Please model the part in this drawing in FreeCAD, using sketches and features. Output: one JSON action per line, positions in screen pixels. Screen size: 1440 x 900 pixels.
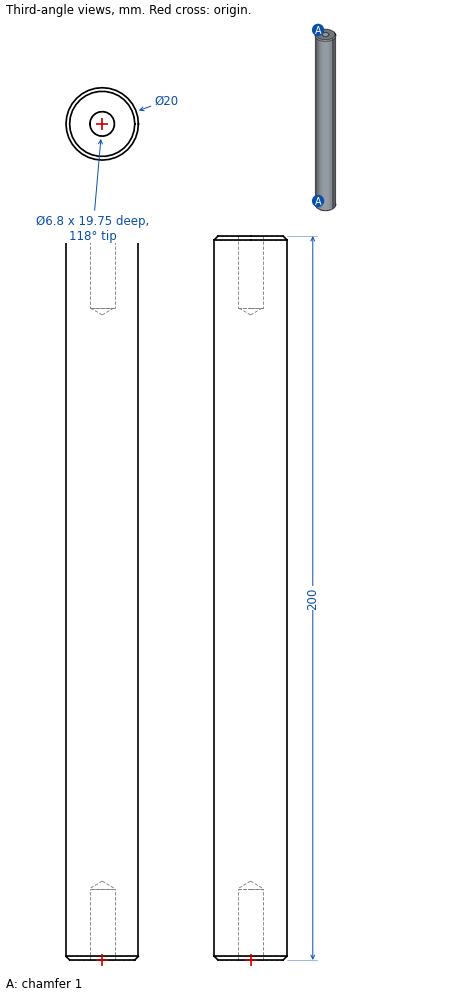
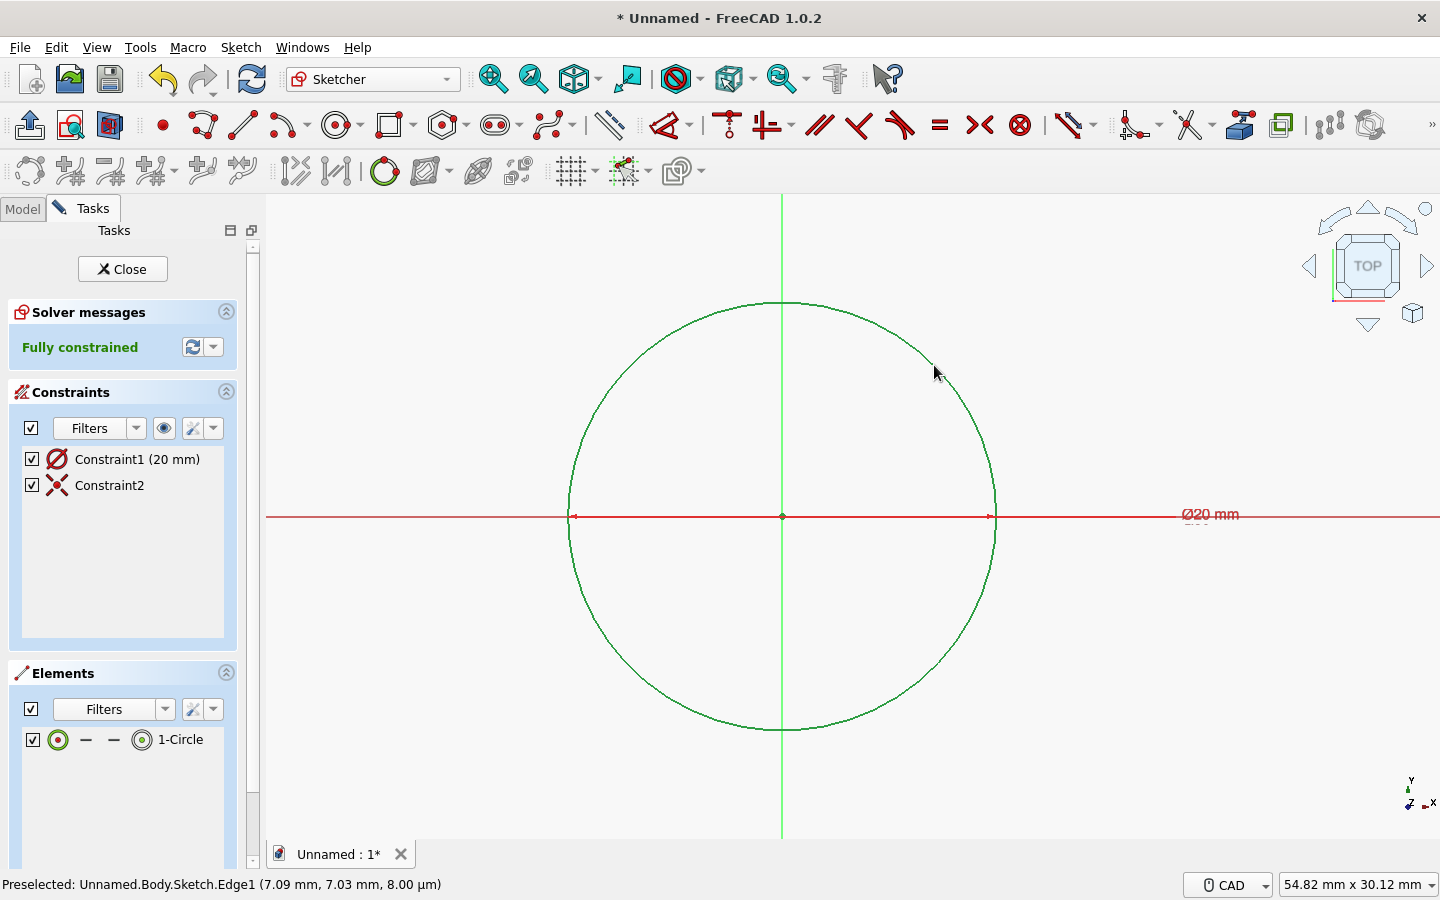
{"action": "left_click", "coordinate": [123, 269]}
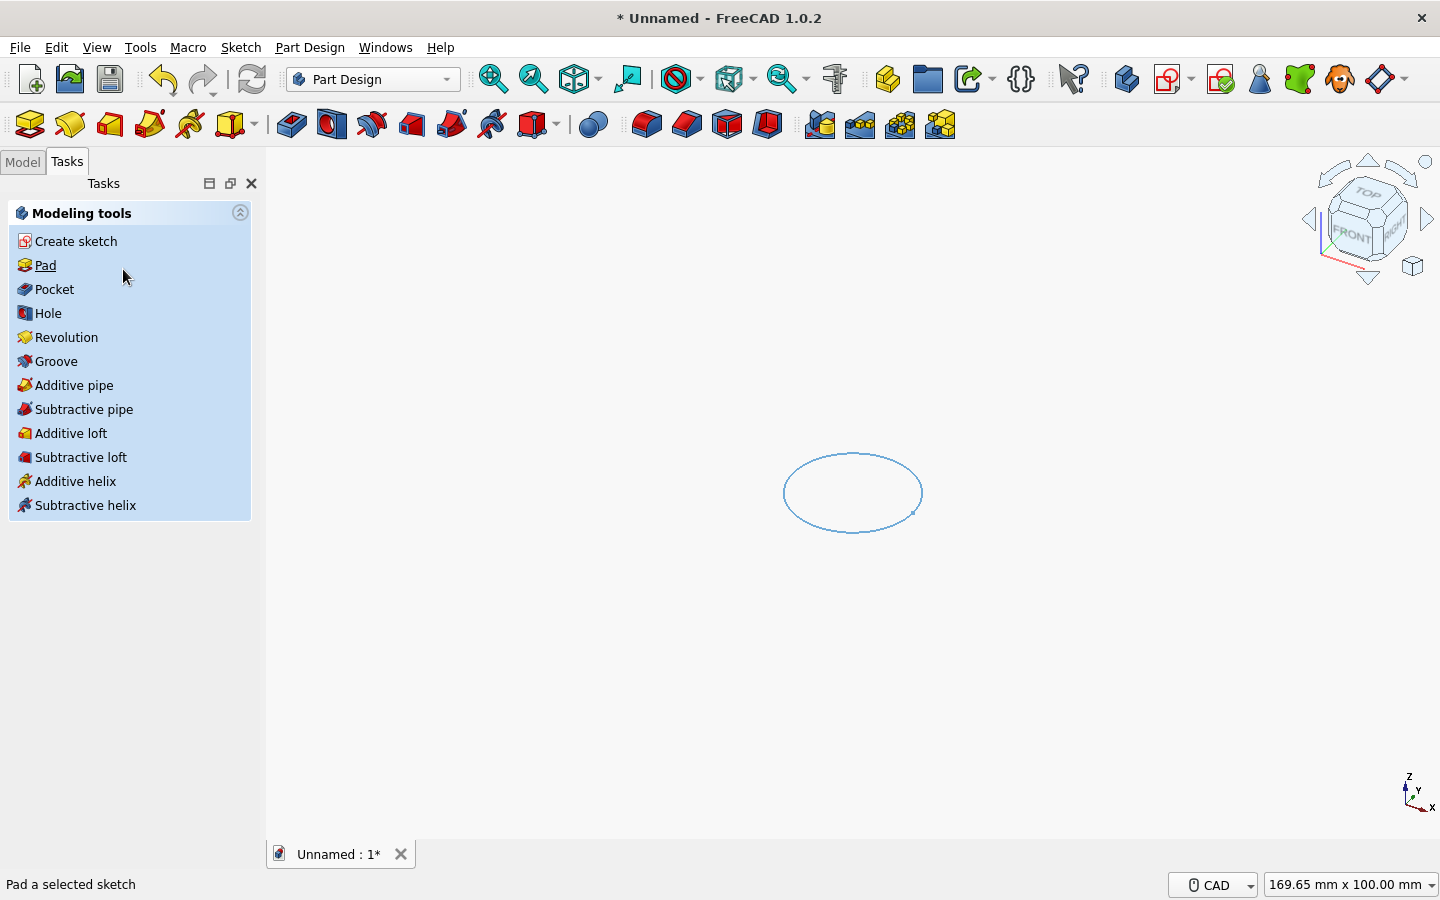
{"action": "left_click", "coordinate": [30, 124]}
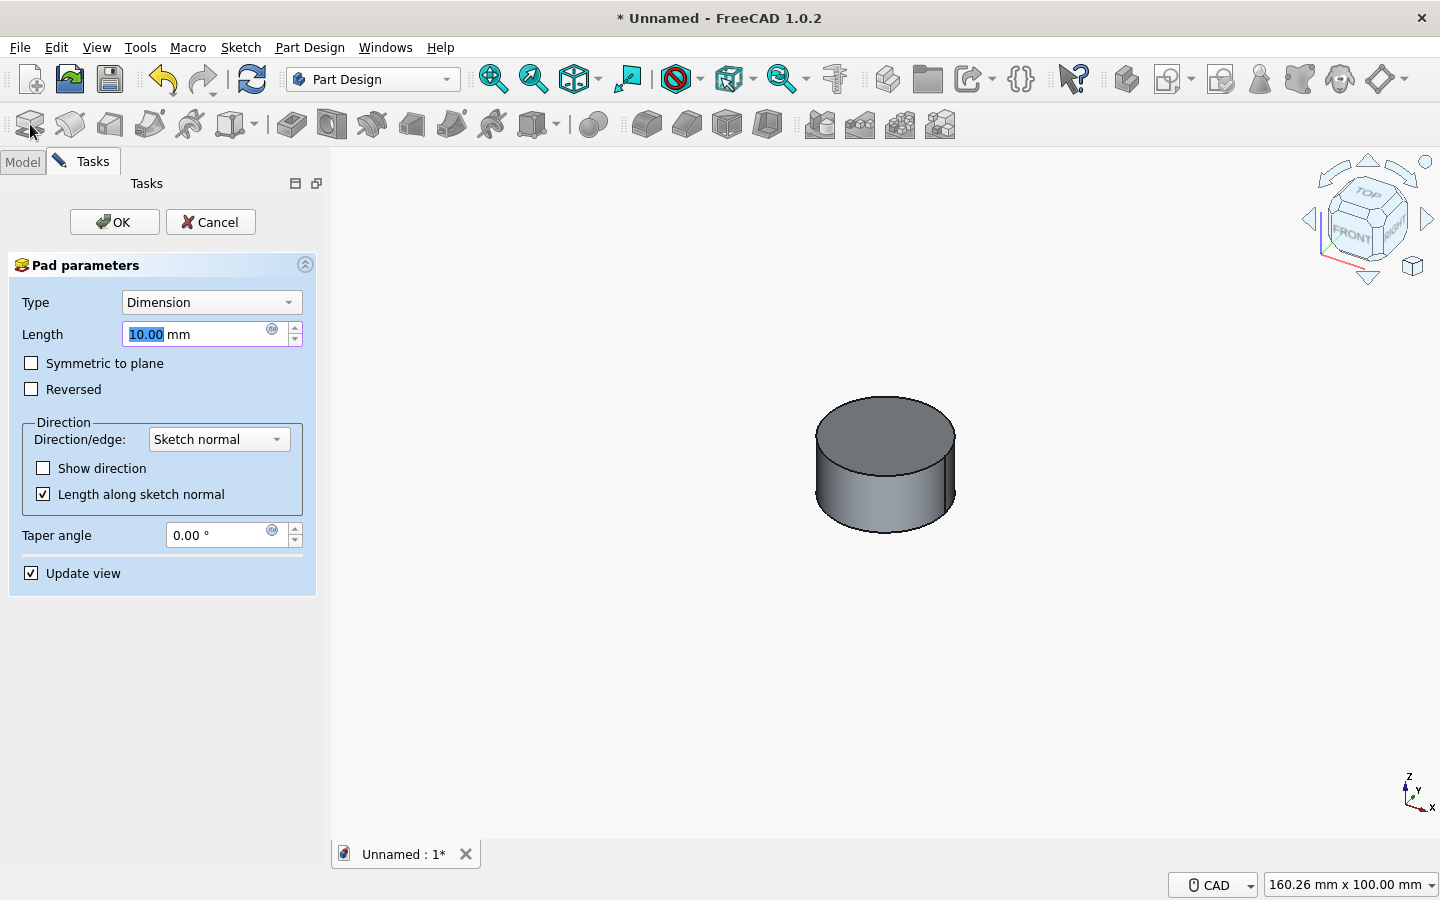
{"action": "type", "text": "200"}
{"action": "key", "text": "Tab"}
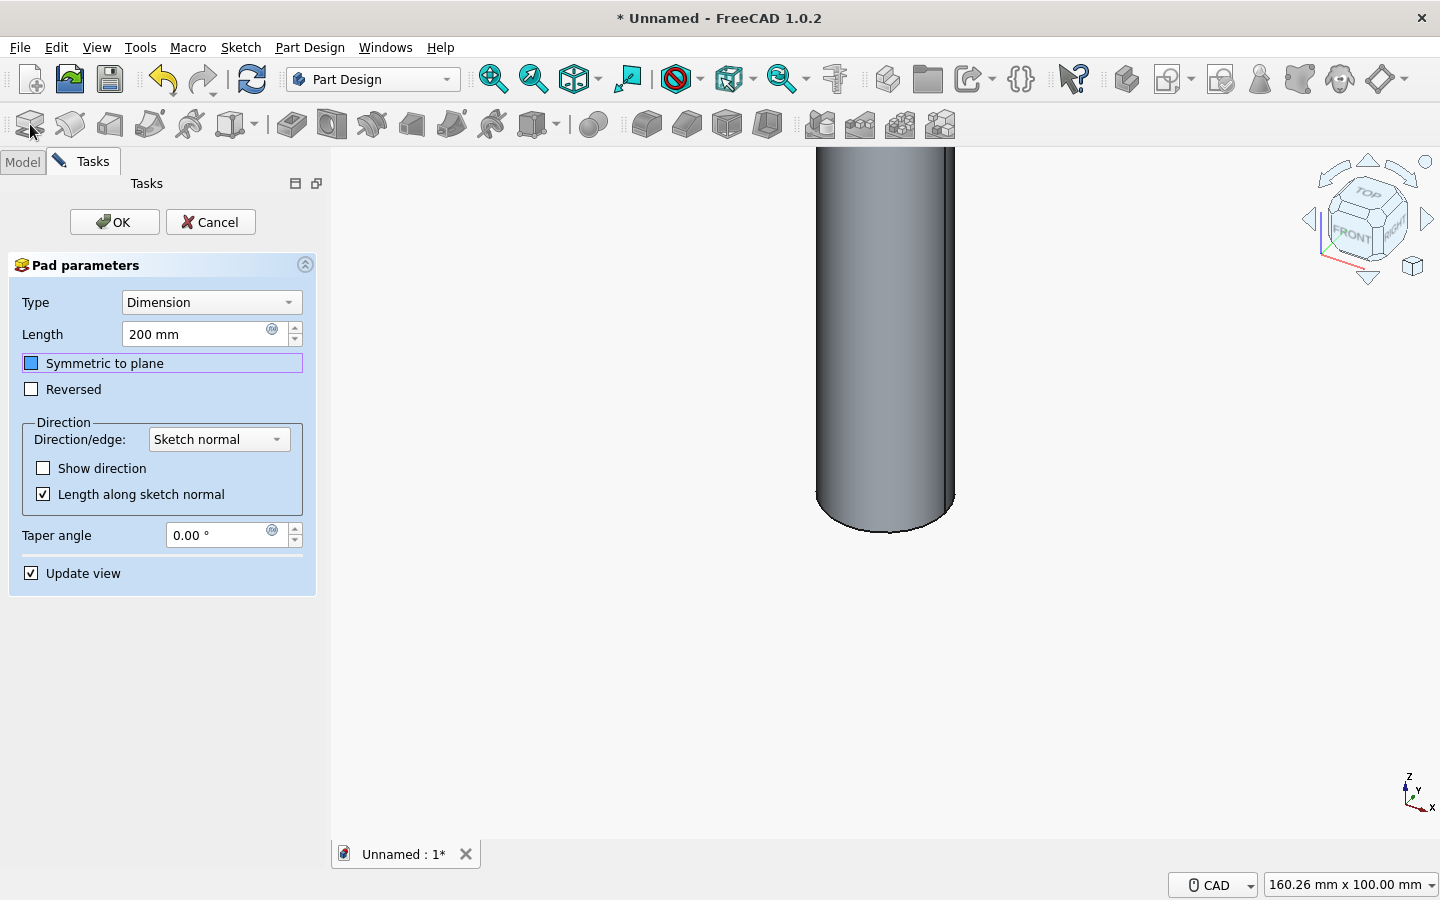
{"action": "left_click", "coordinate": [115, 222]}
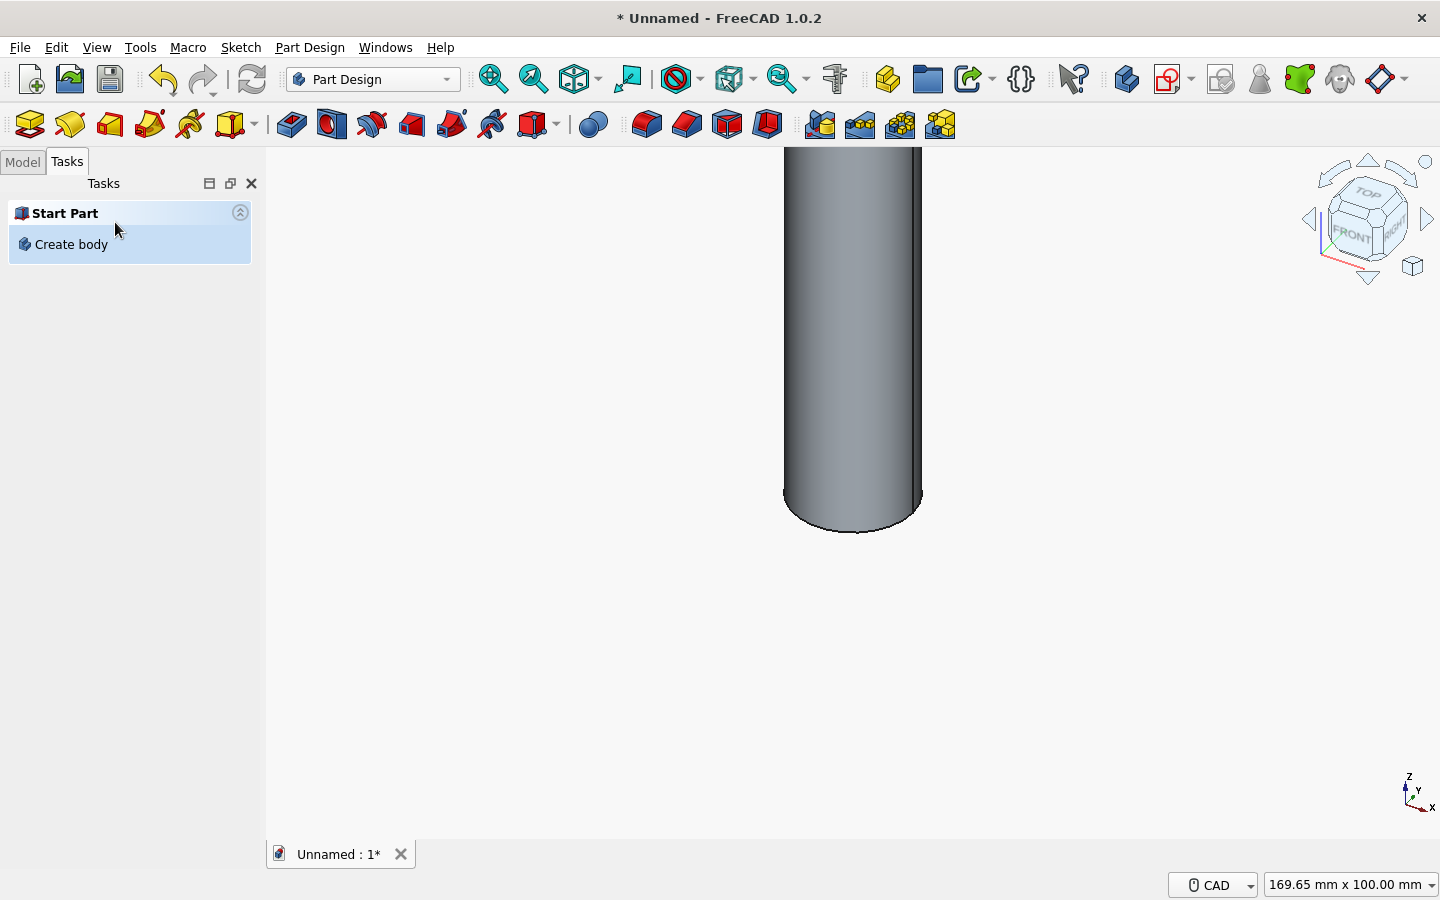
{"action": "left_click", "coordinate": [494, 80]}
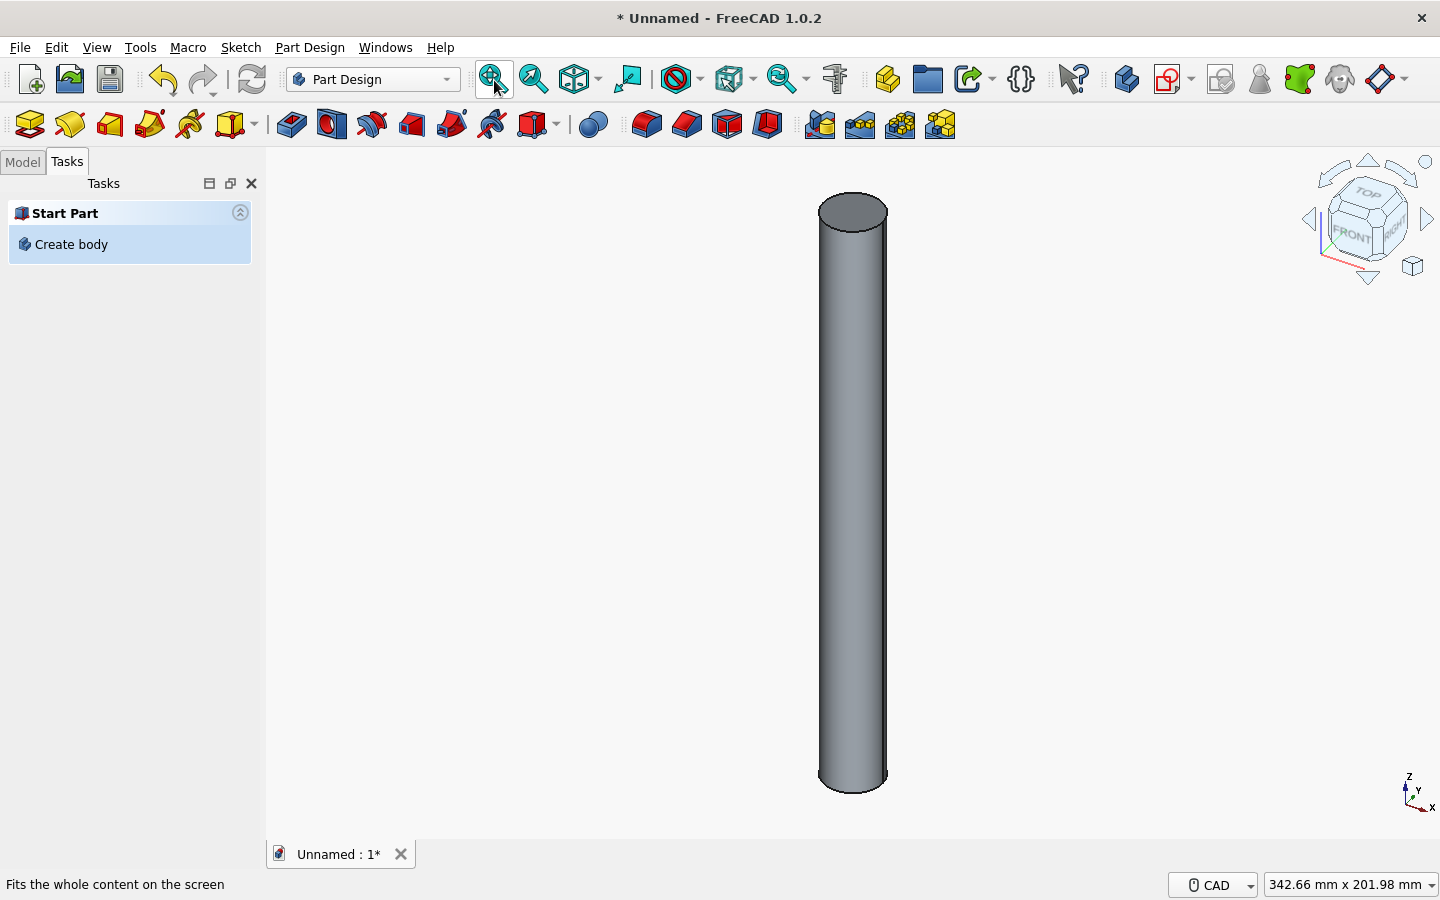
{"action": "key", "text": "5"}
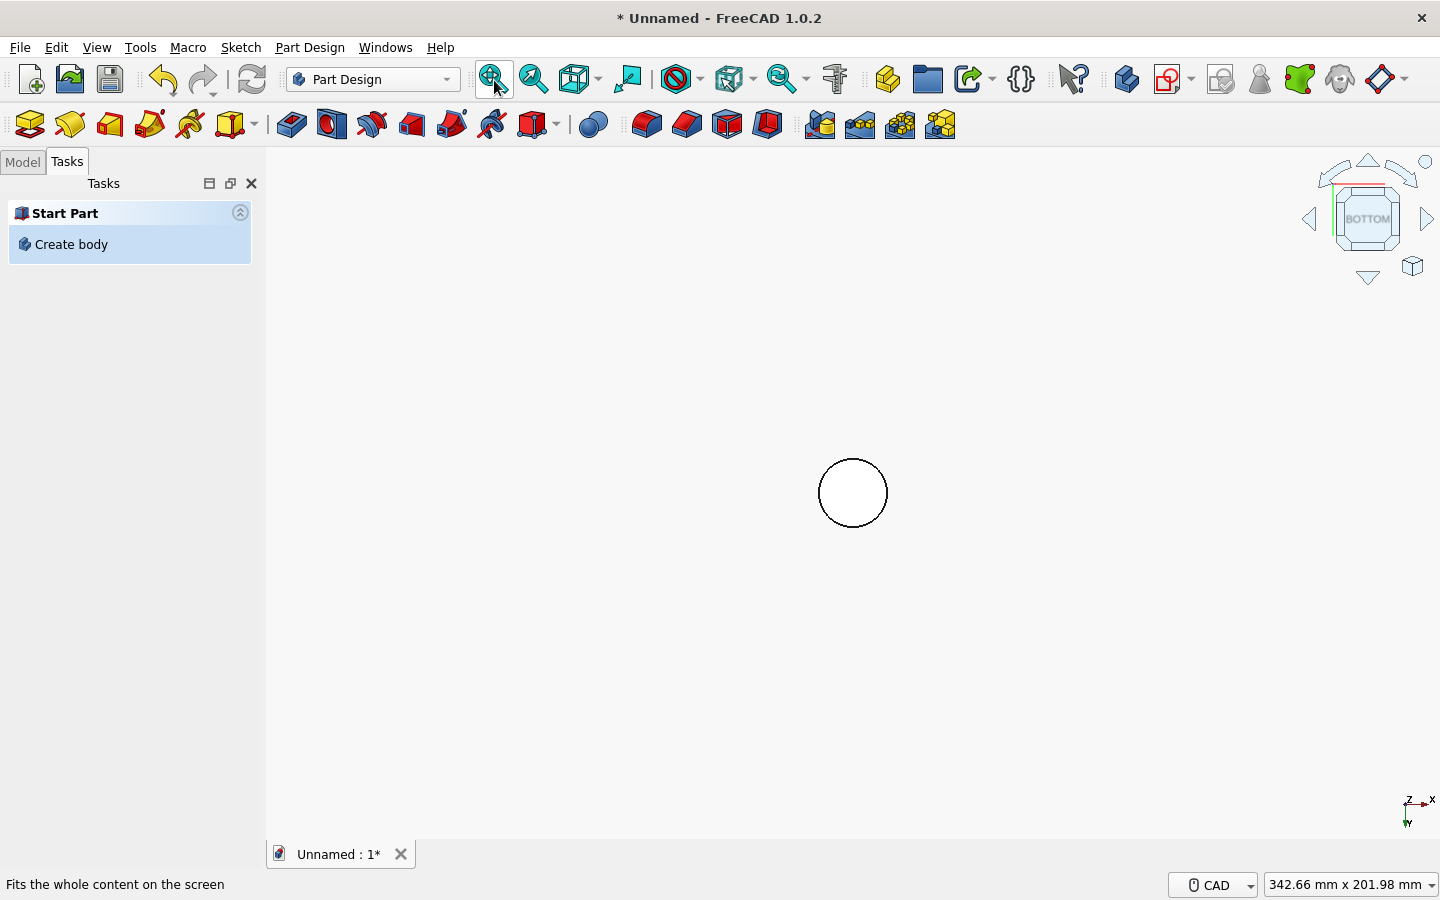
{"action": "left_click", "coordinate": [494, 80]}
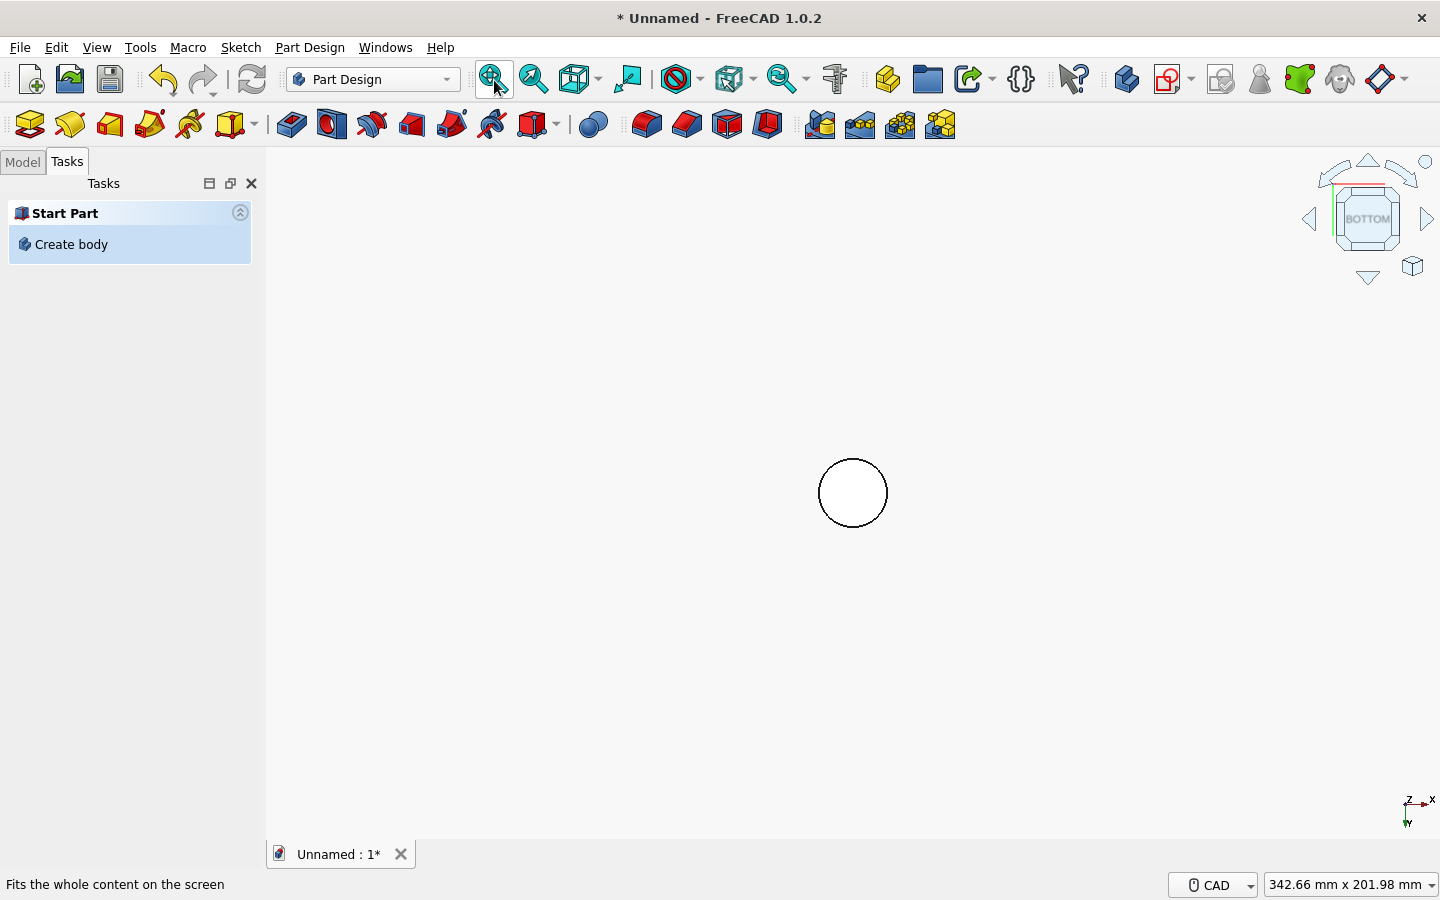
{"action": "left_click", "coordinate": [853, 492]}